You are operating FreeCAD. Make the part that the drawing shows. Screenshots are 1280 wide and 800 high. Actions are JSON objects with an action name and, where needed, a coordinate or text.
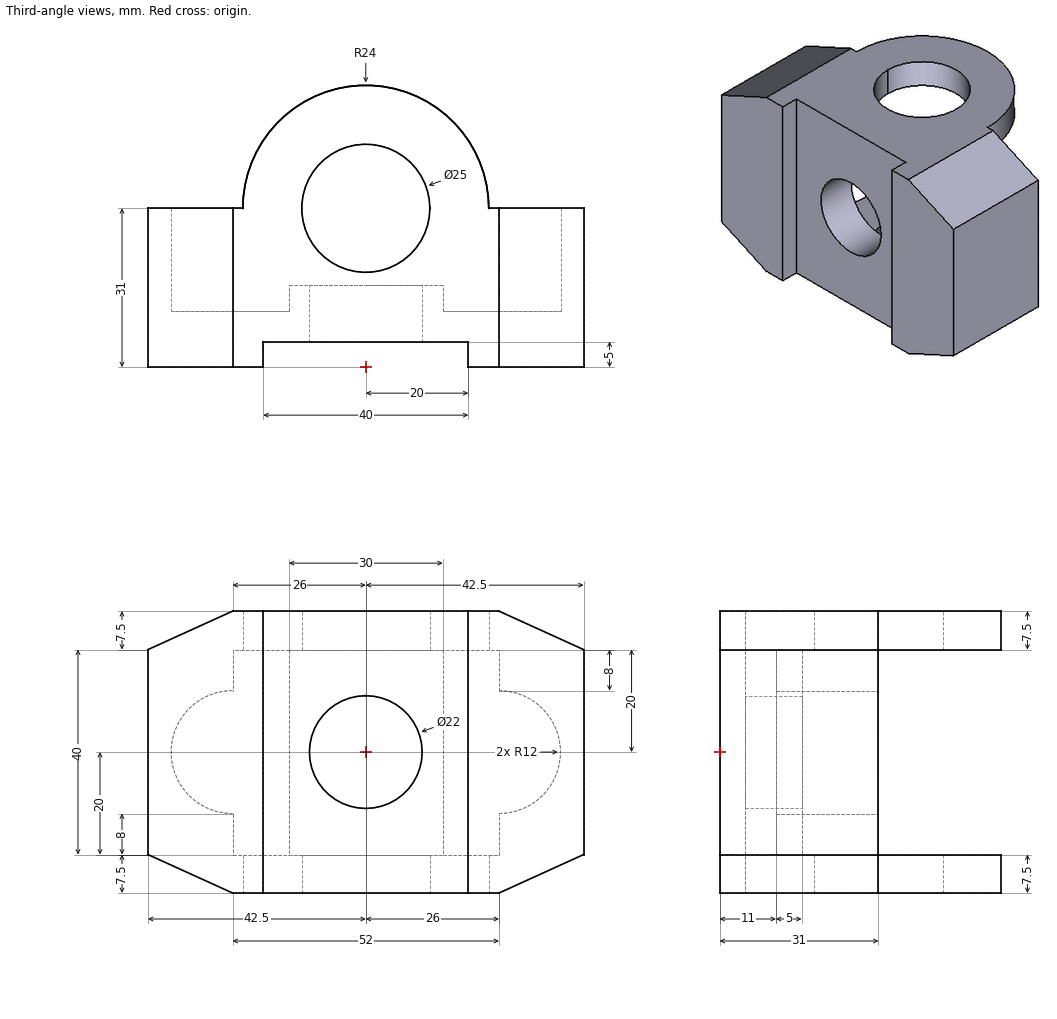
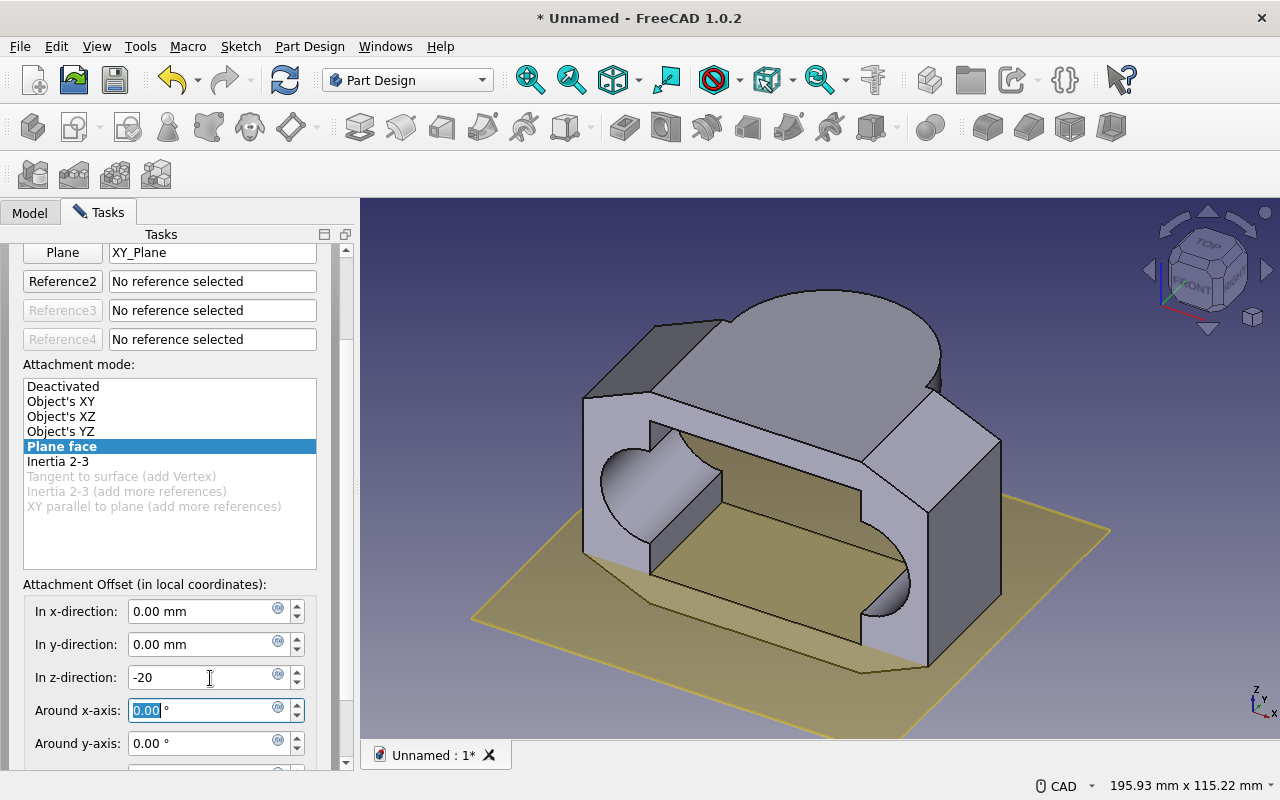
{"action": "scroll", "coordinate": [346, 507], "scroll_direction": "up", "scroll_amount": 3}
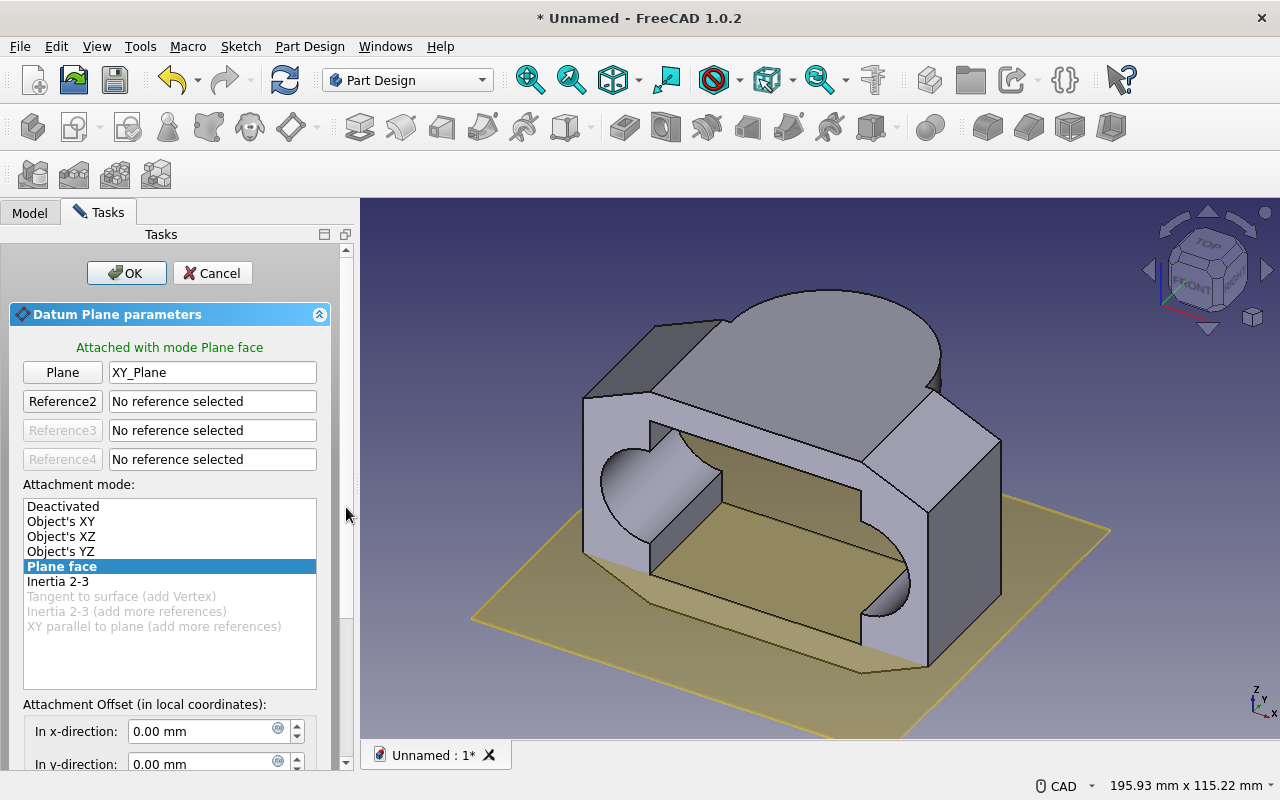
{"action": "left_click", "coordinate": [127, 273]}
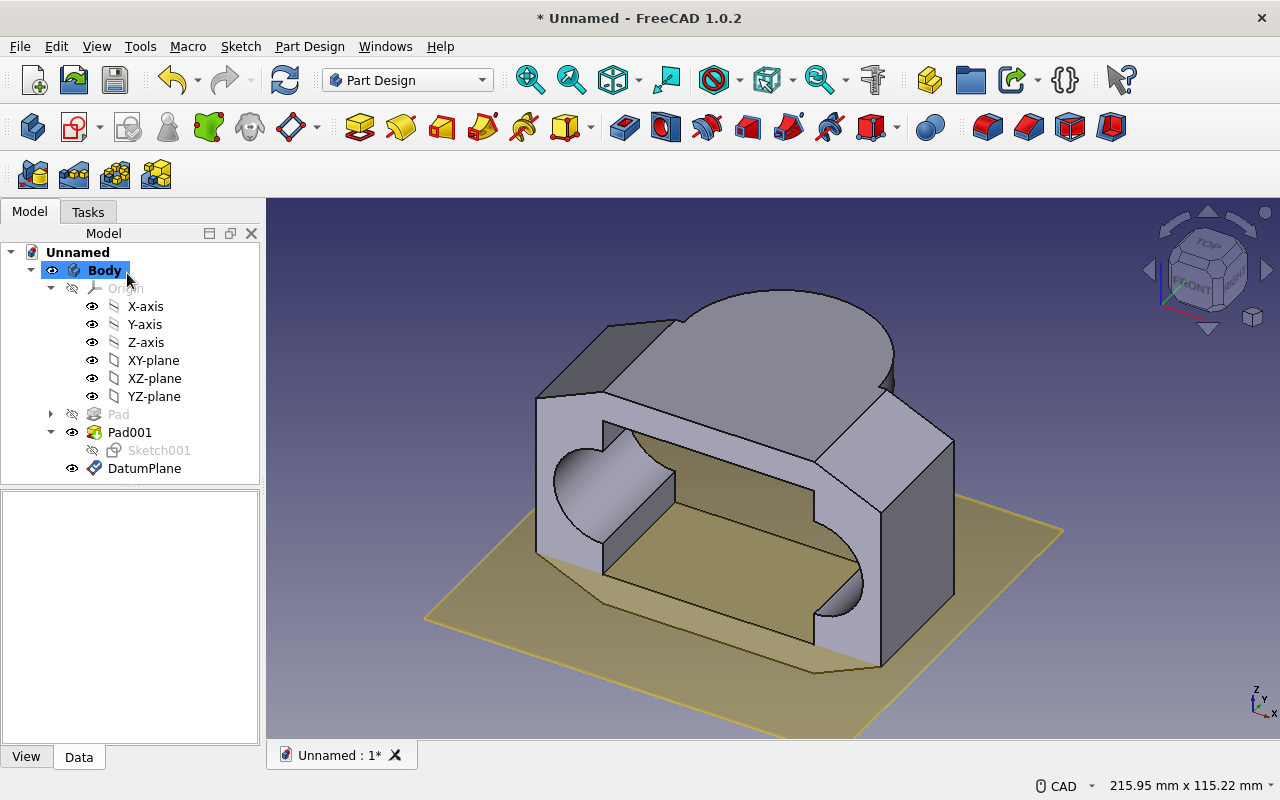
{"action": "left_click", "coordinate": [117, 468]}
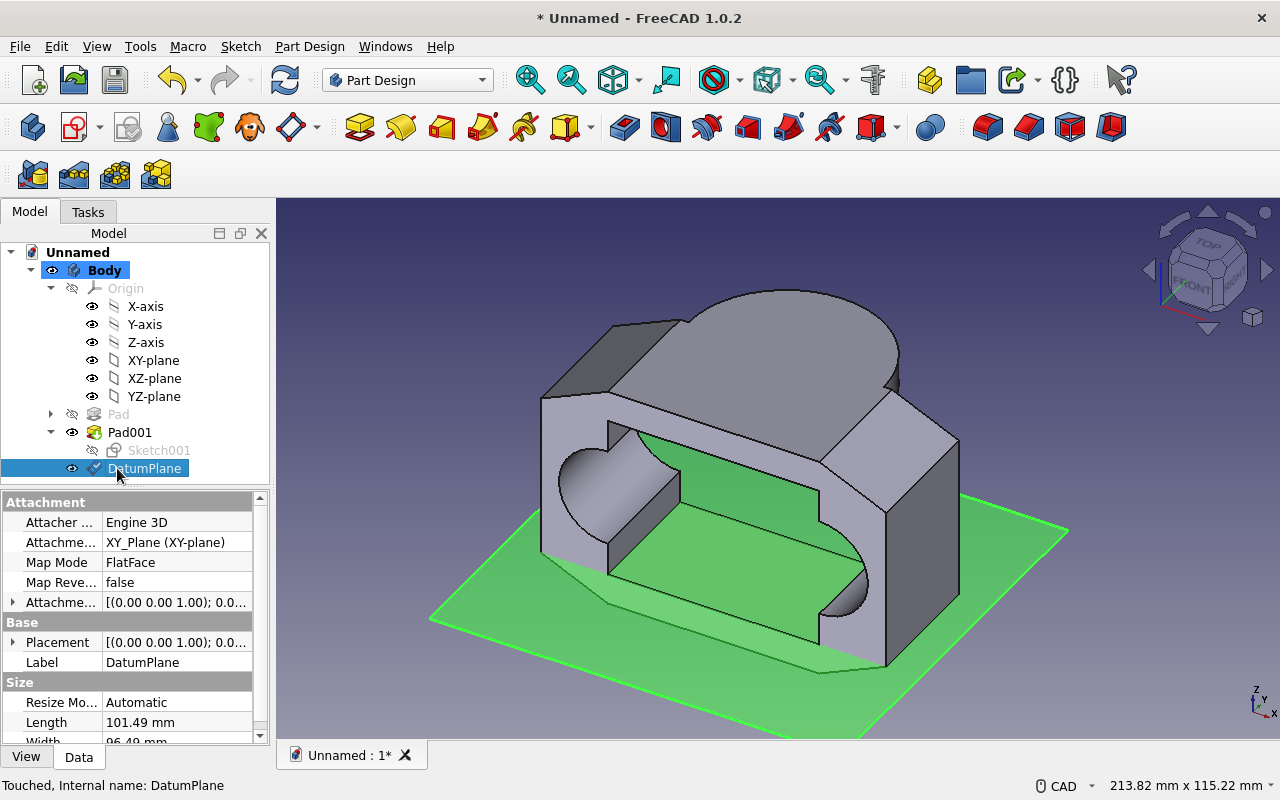
{"action": "left_click", "coordinate": [74, 128]}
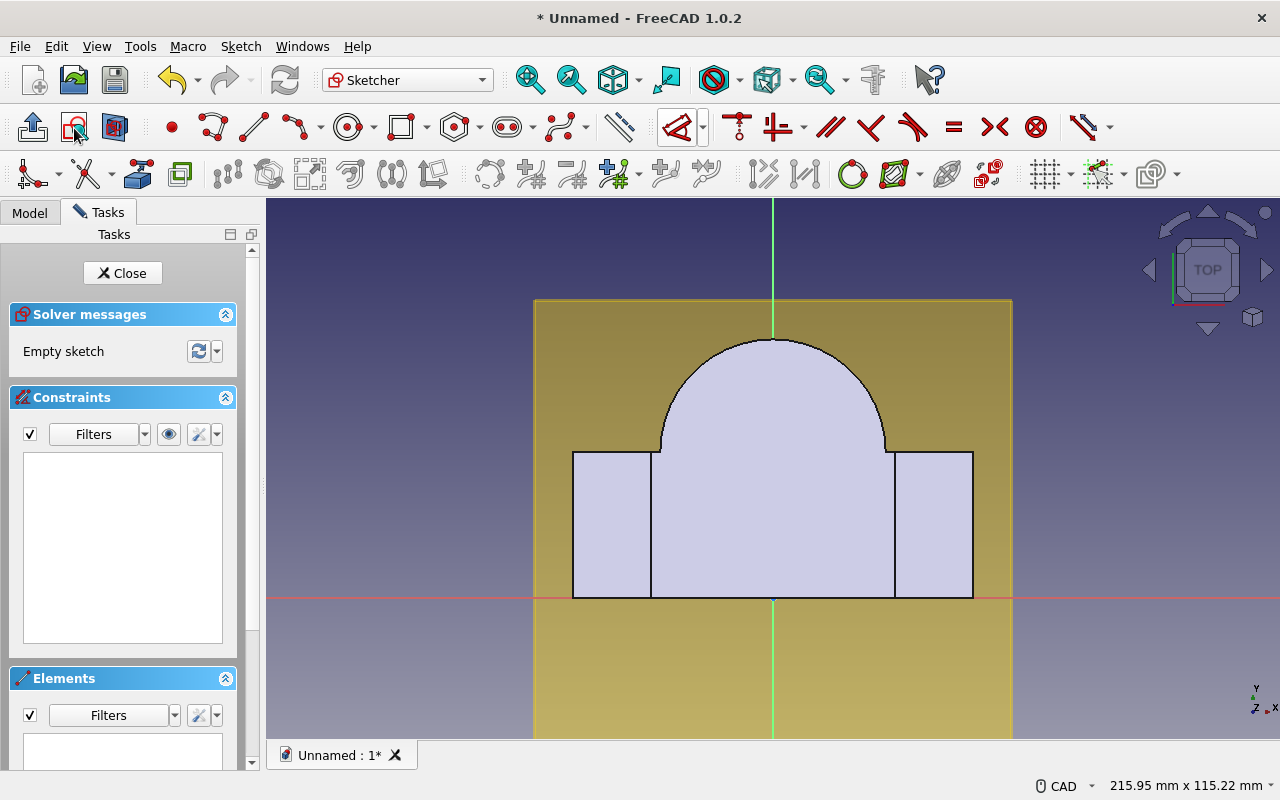
{"action": "left_click", "coordinate": [115, 128]}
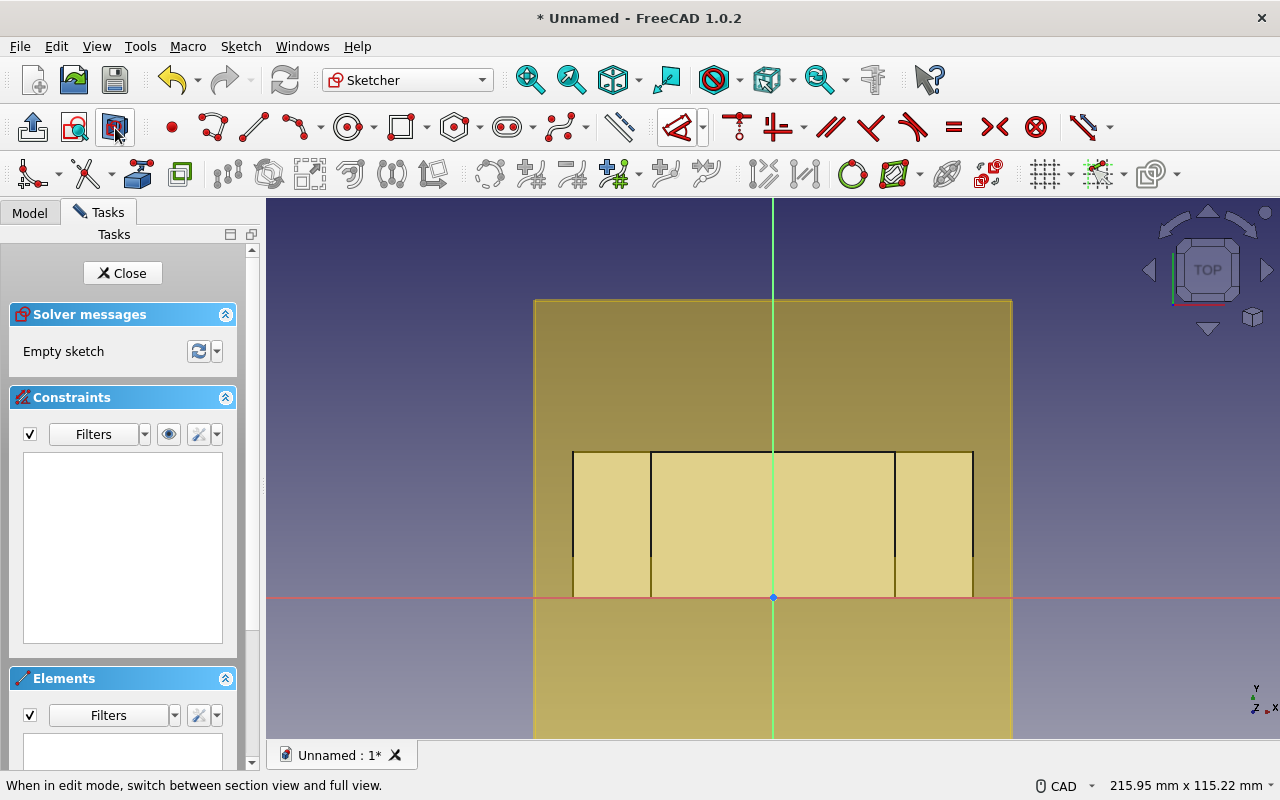
{"action": "left_click", "coordinate": [254, 128]}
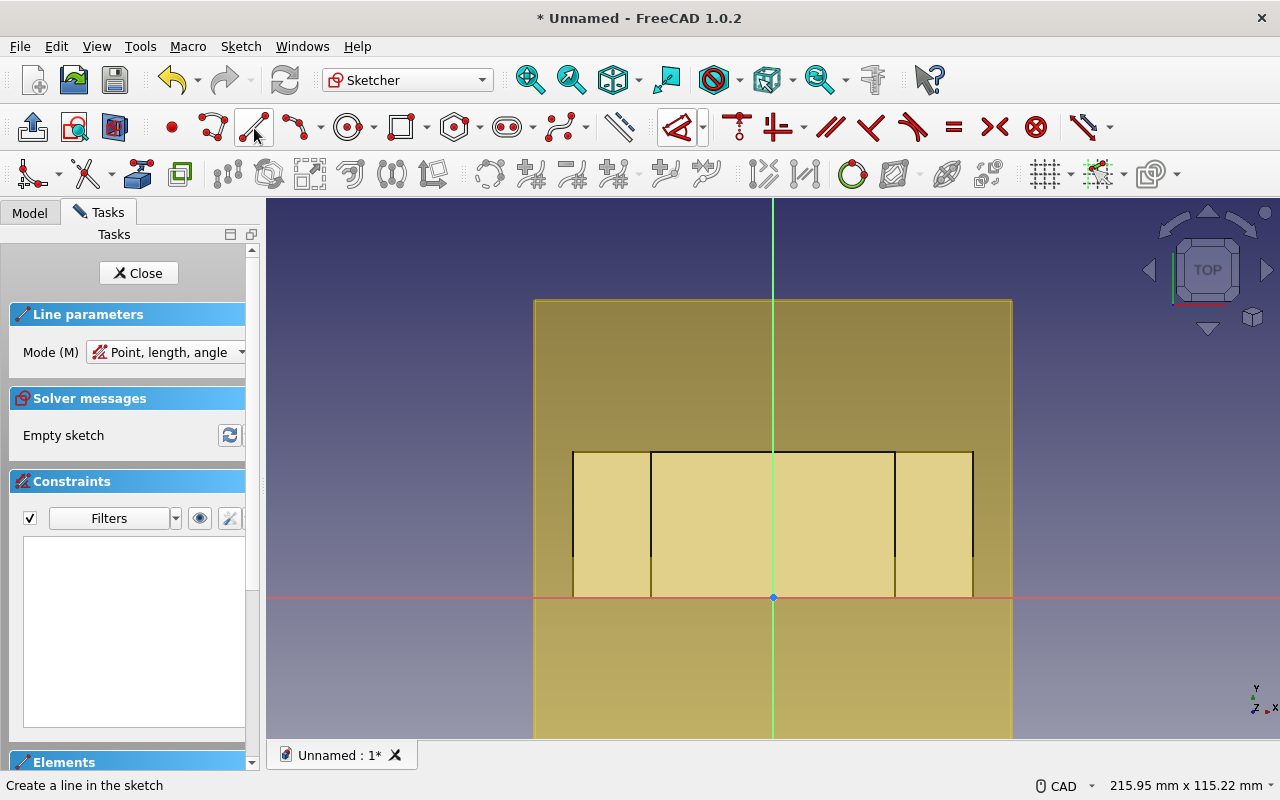
{"action": "left_click", "coordinate": [886, 452]}
{"action": "left_click", "coordinate": [660, 452]}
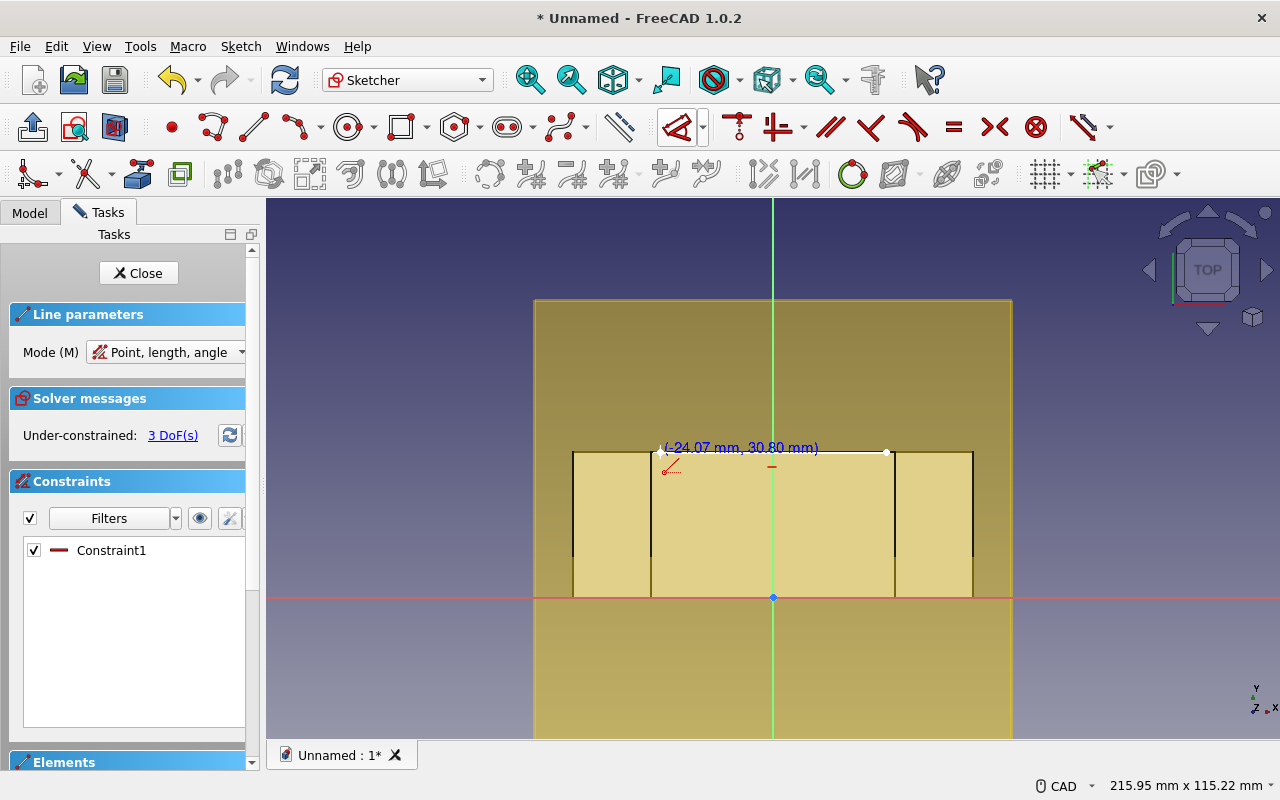
{"action": "key", "text": "g 3 a"}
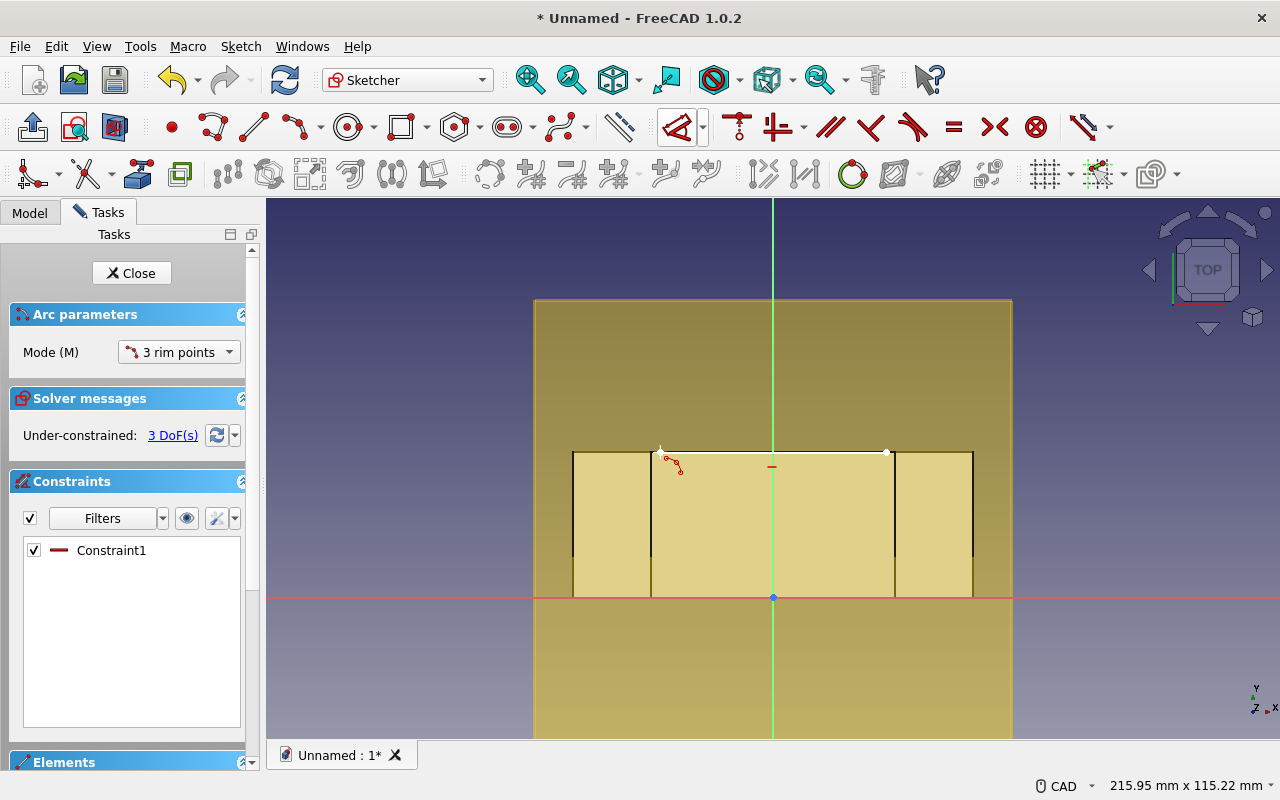
{"action": "left_click", "coordinate": [660, 453]}
{"action": "left_click", "coordinate": [886, 453]}
{"action": "left_click", "coordinate": [808, 345]}
{"action": "key", "text": "Escape"}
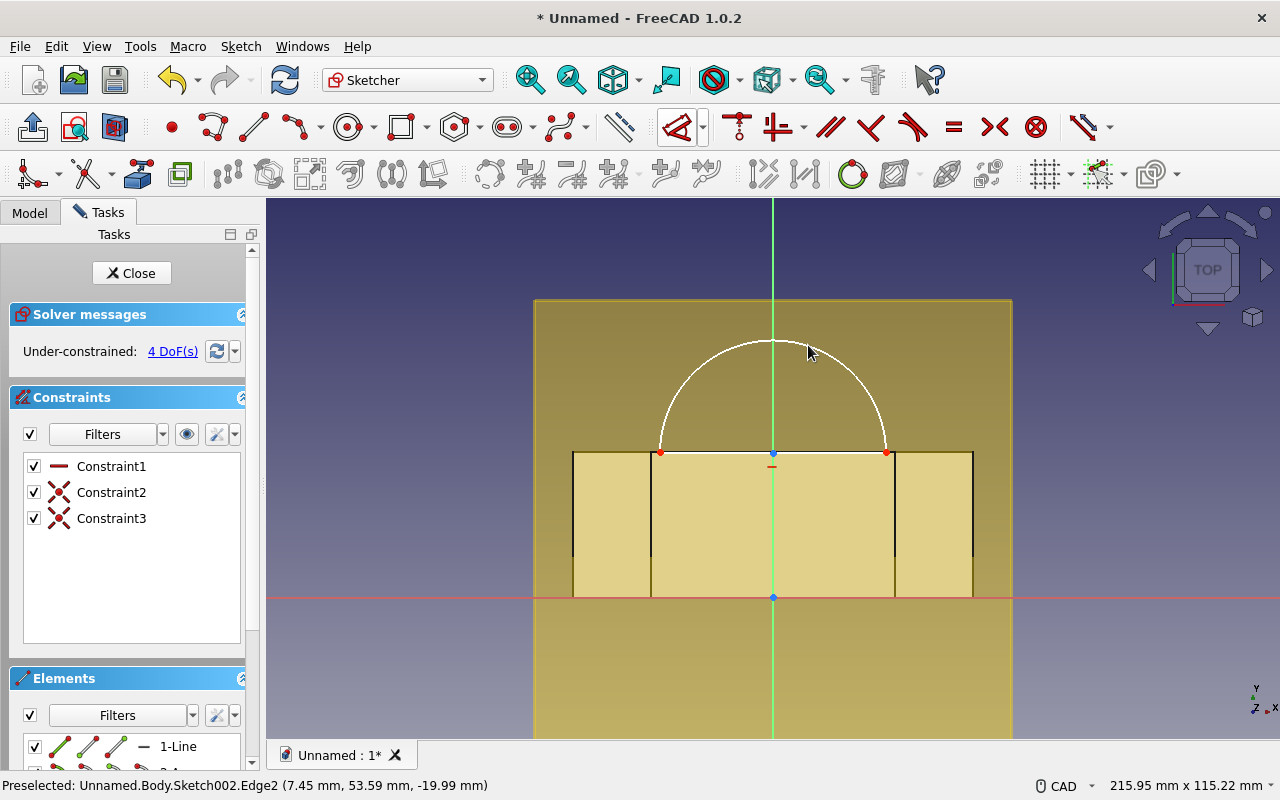
{"action": "left_click", "coordinate": [773, 453]}